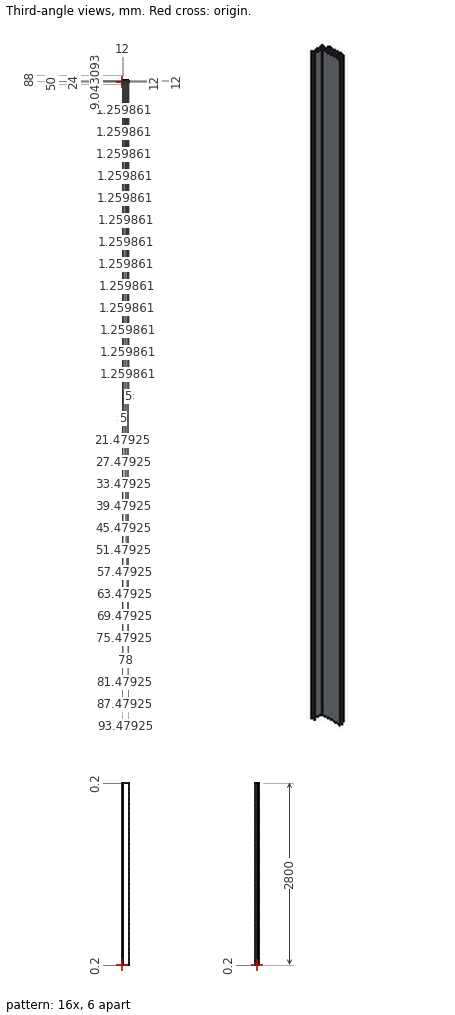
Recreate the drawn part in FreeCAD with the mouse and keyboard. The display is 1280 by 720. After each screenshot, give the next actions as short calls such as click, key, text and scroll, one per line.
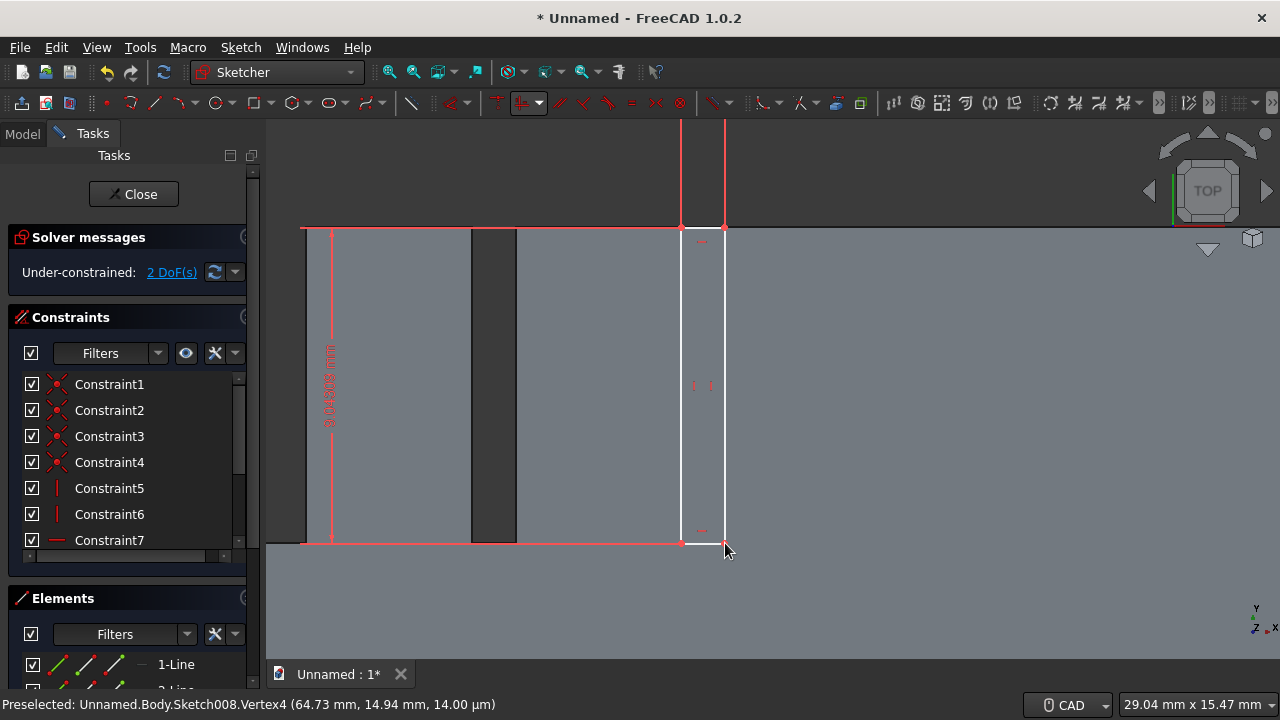
click(450, 104)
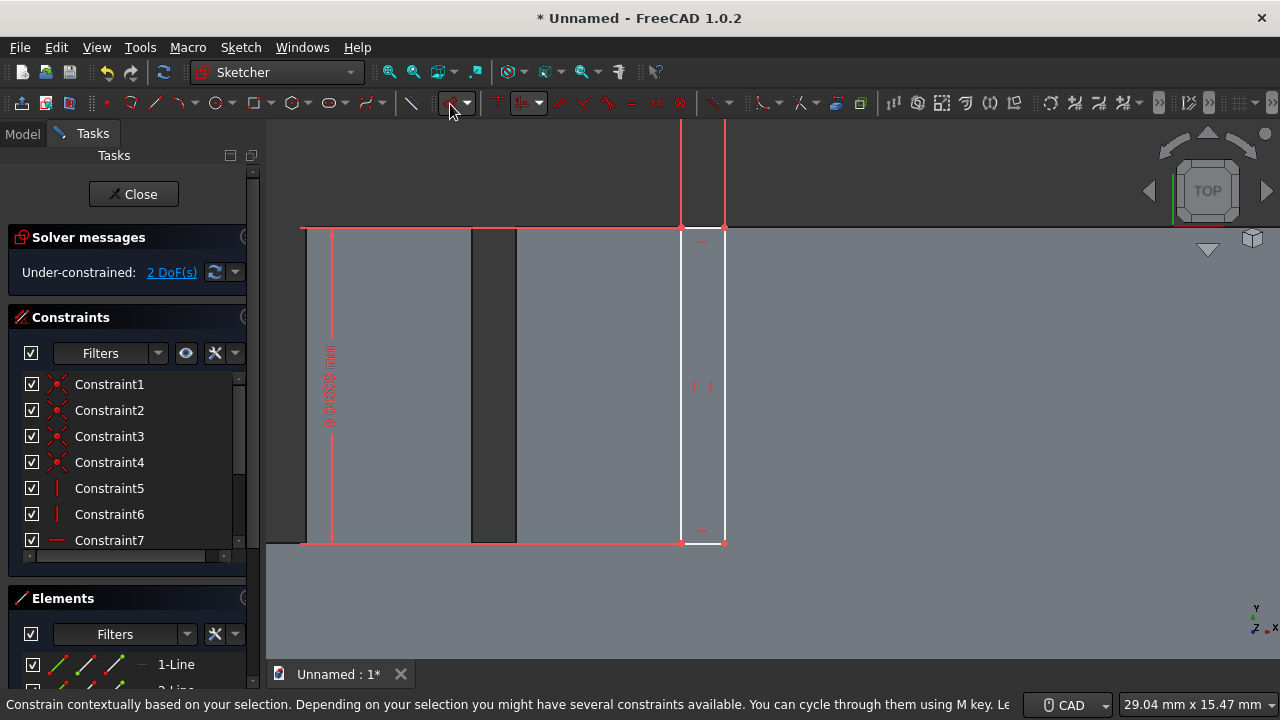
click(681, 228)
click(715, 571)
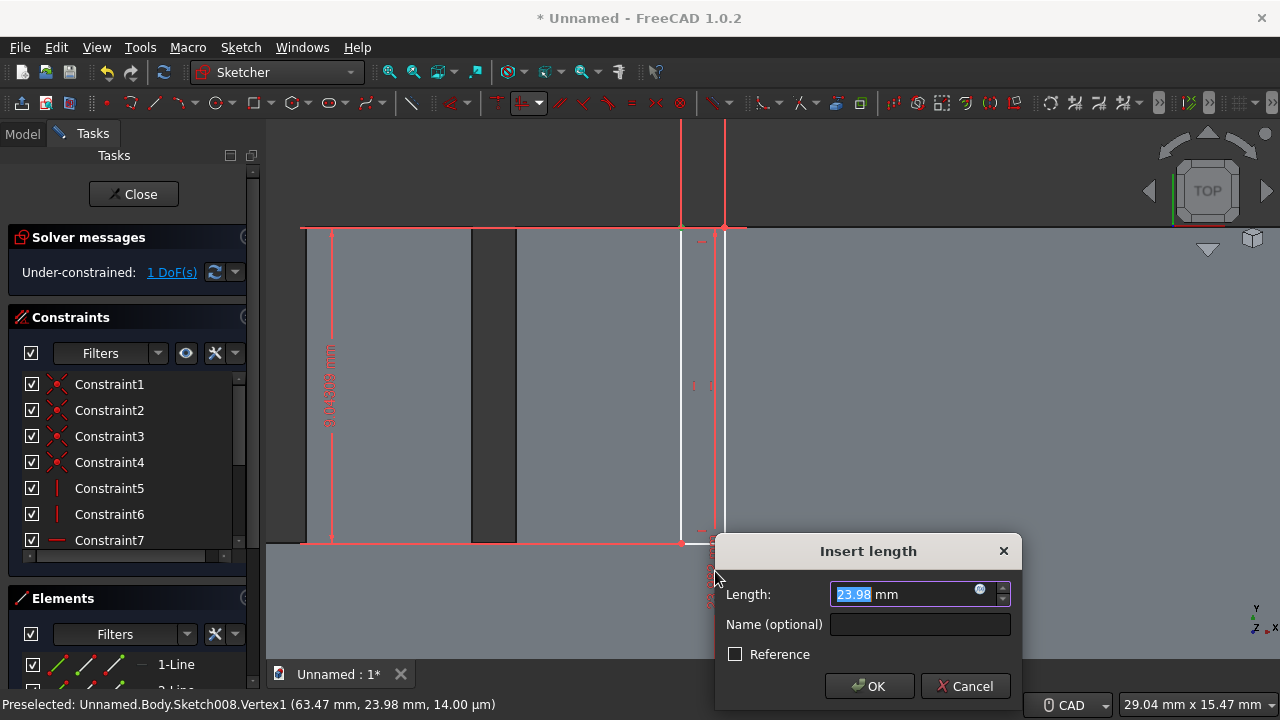
text(24)
key(Return)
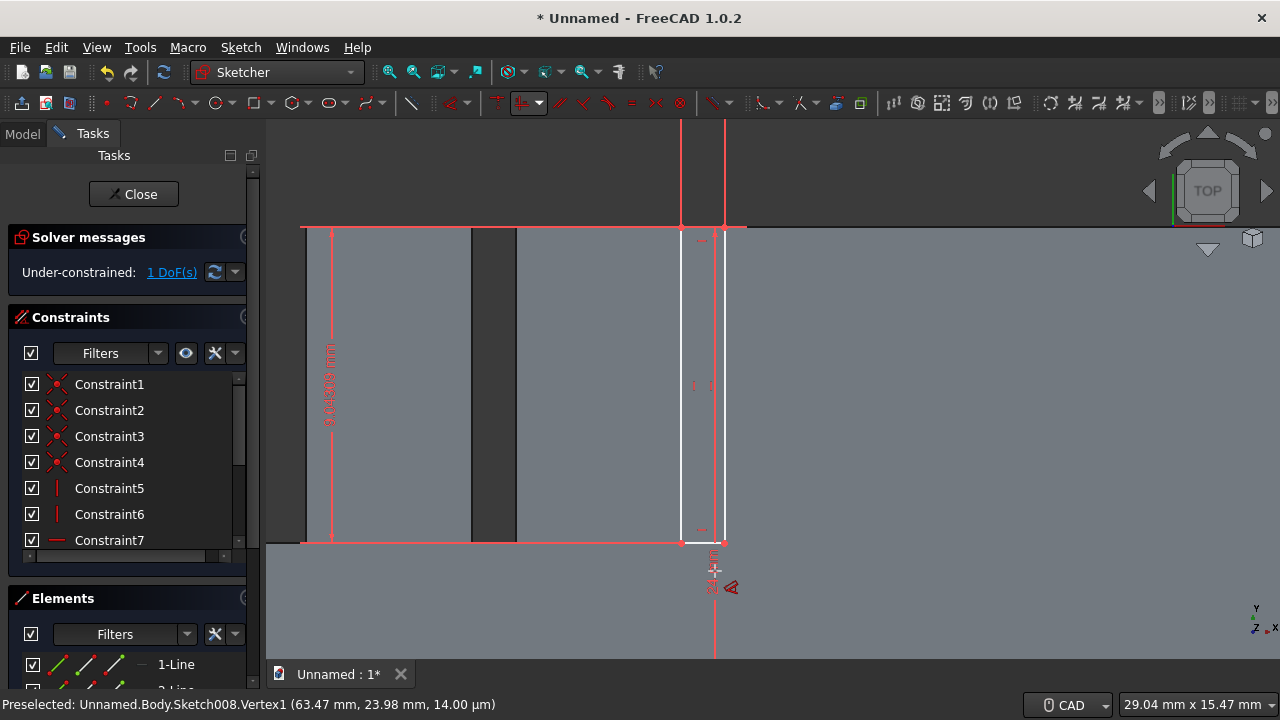
click(681, 227)
click(488, 193)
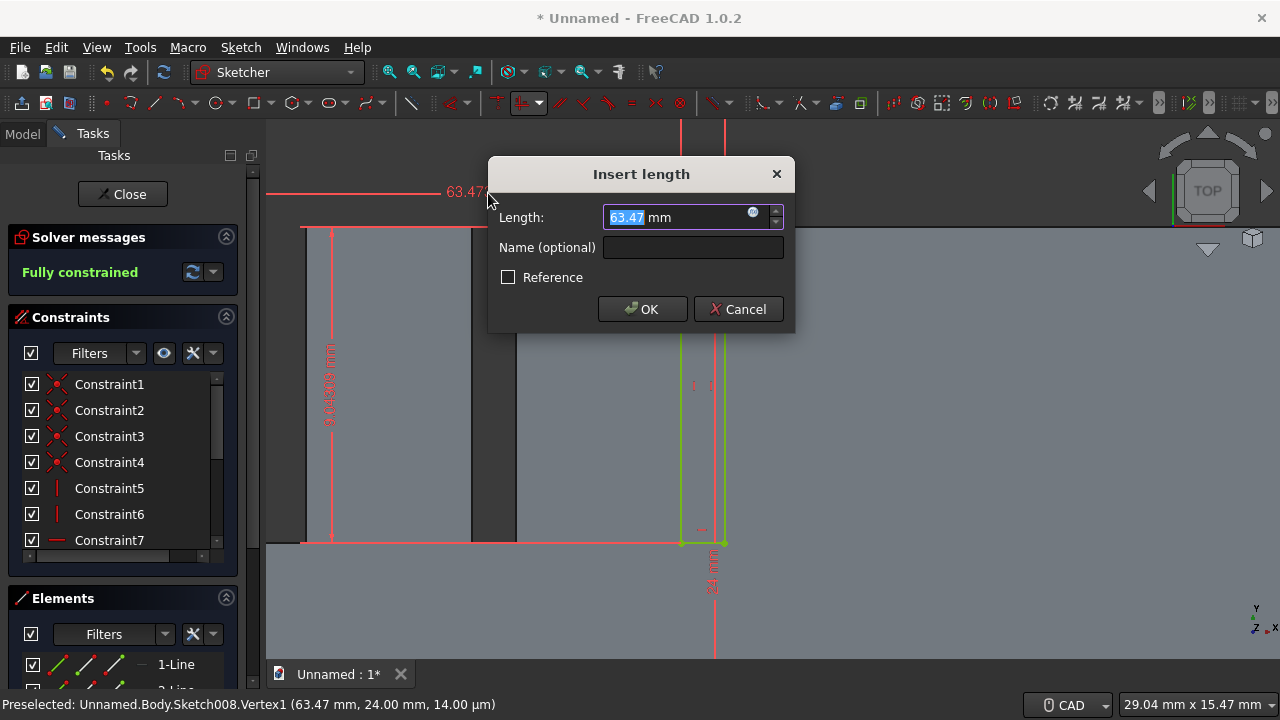
text(63.47925)
key(Return)
key(Escape)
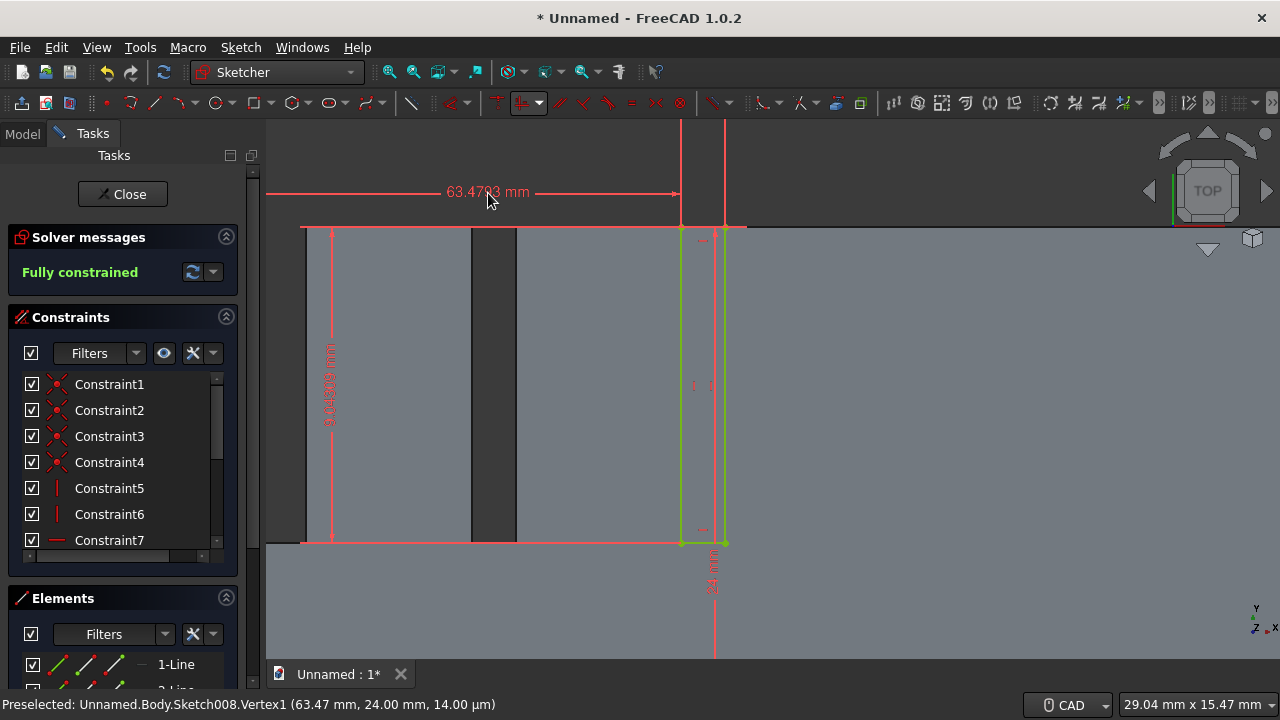
click(123, 194)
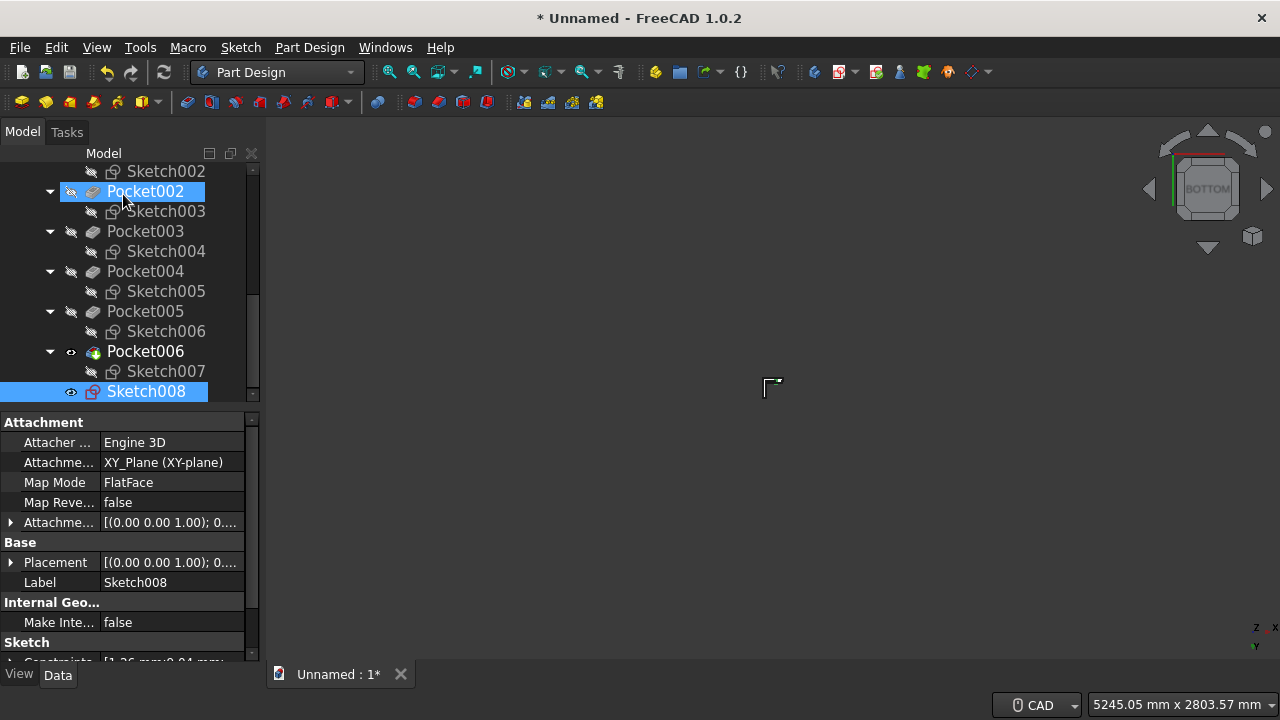
click(188, 102)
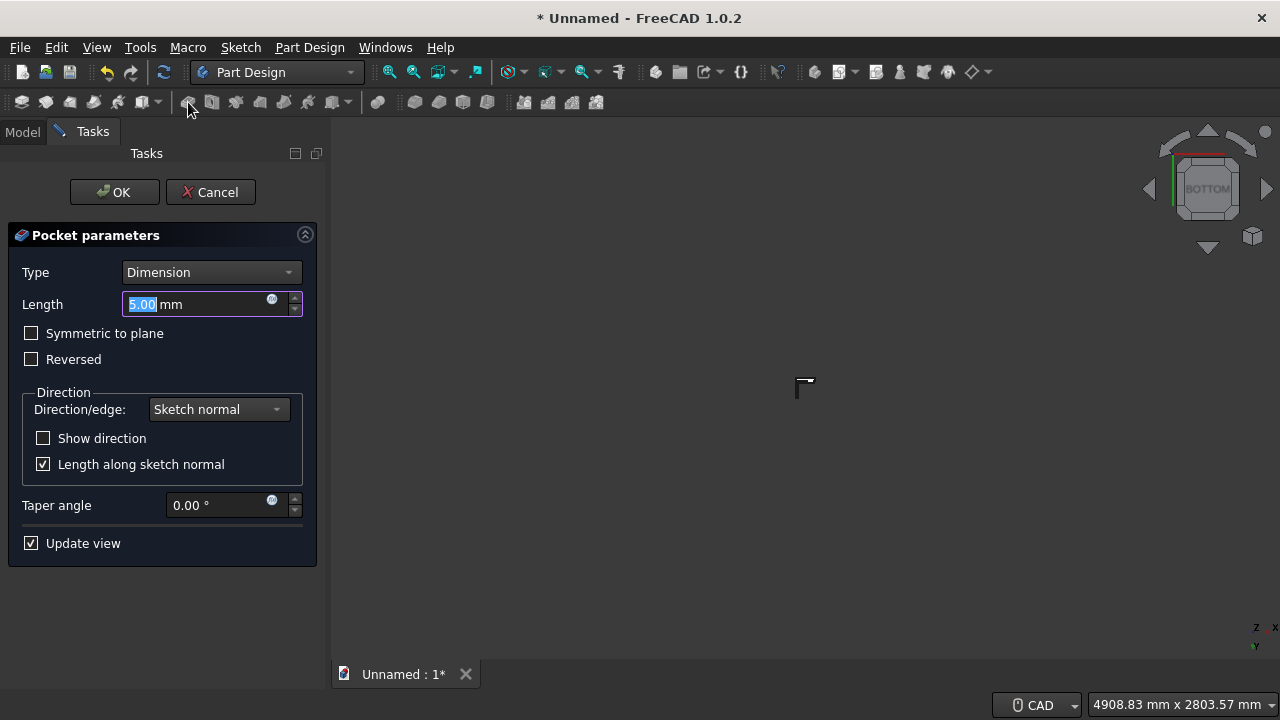
text(0.2)
key(Tab)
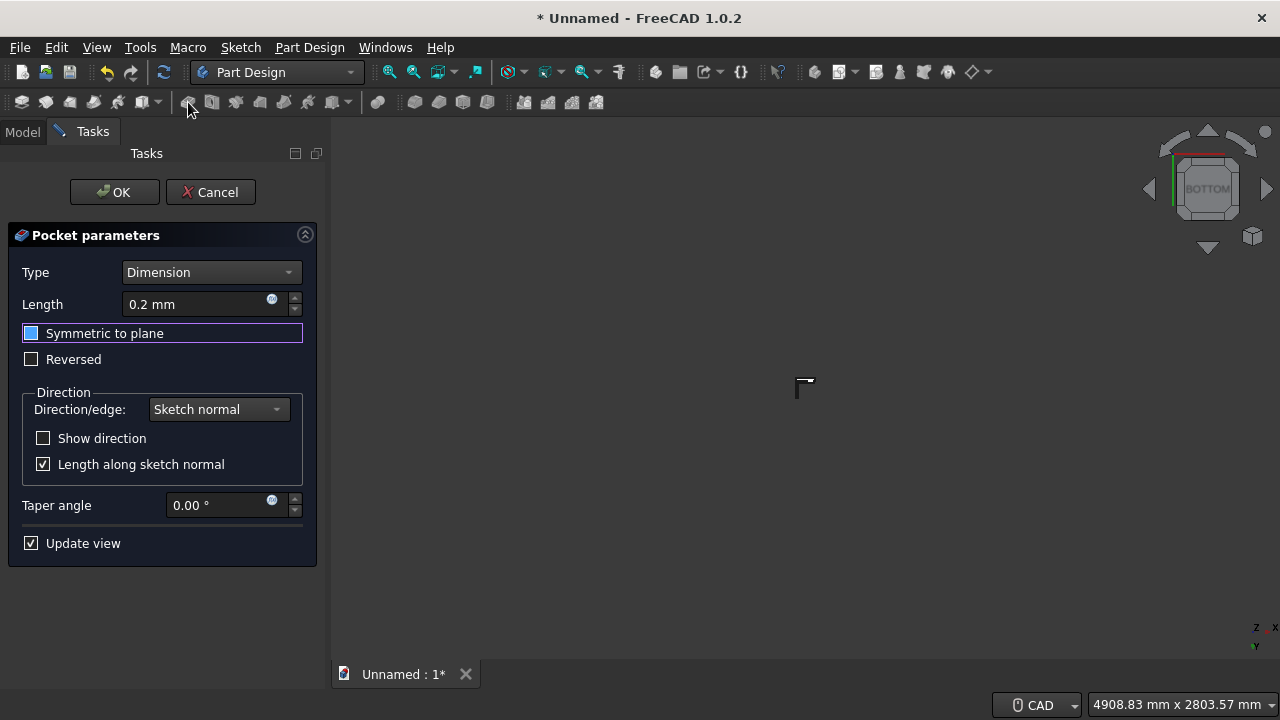
click(30, 359)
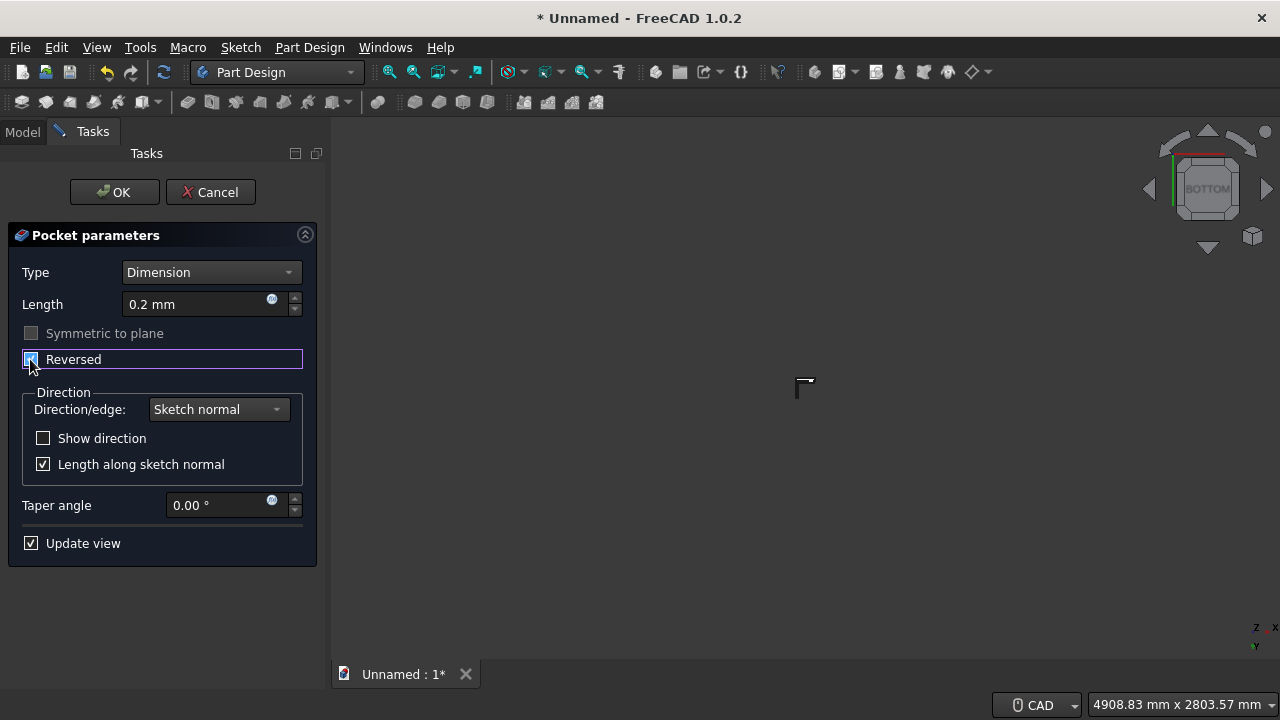
click(115, 192)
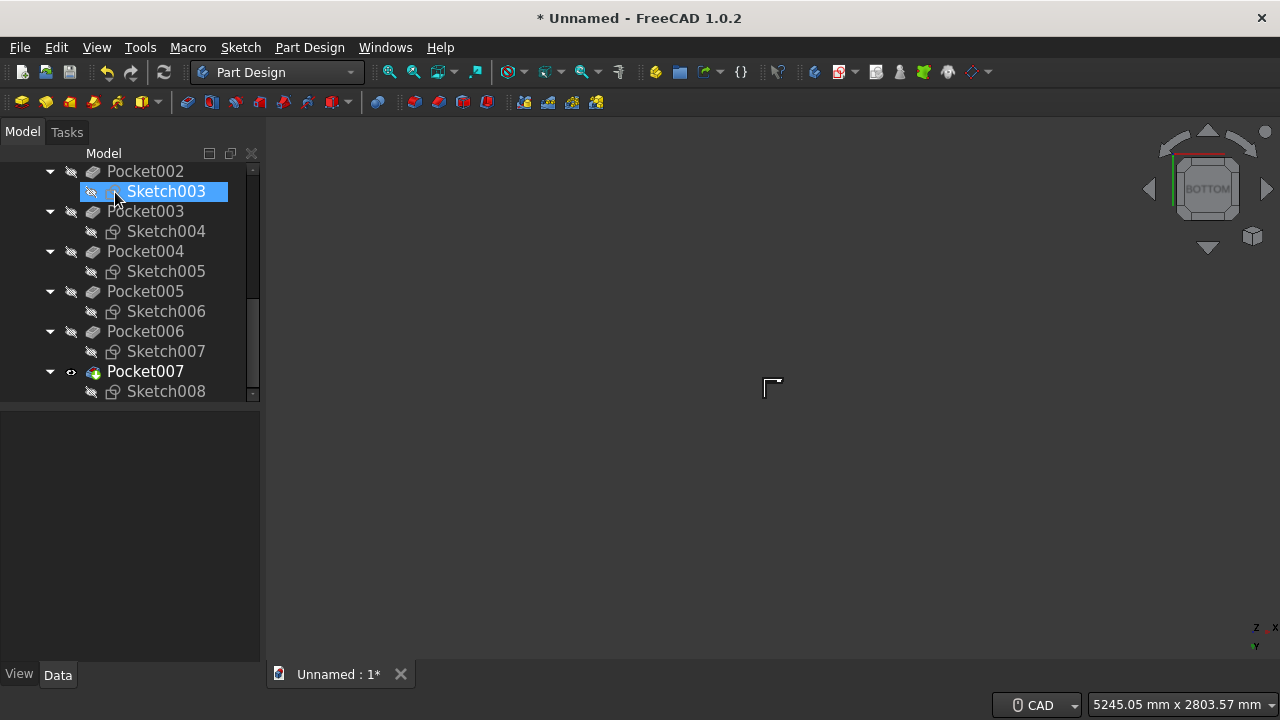
click(390, 72)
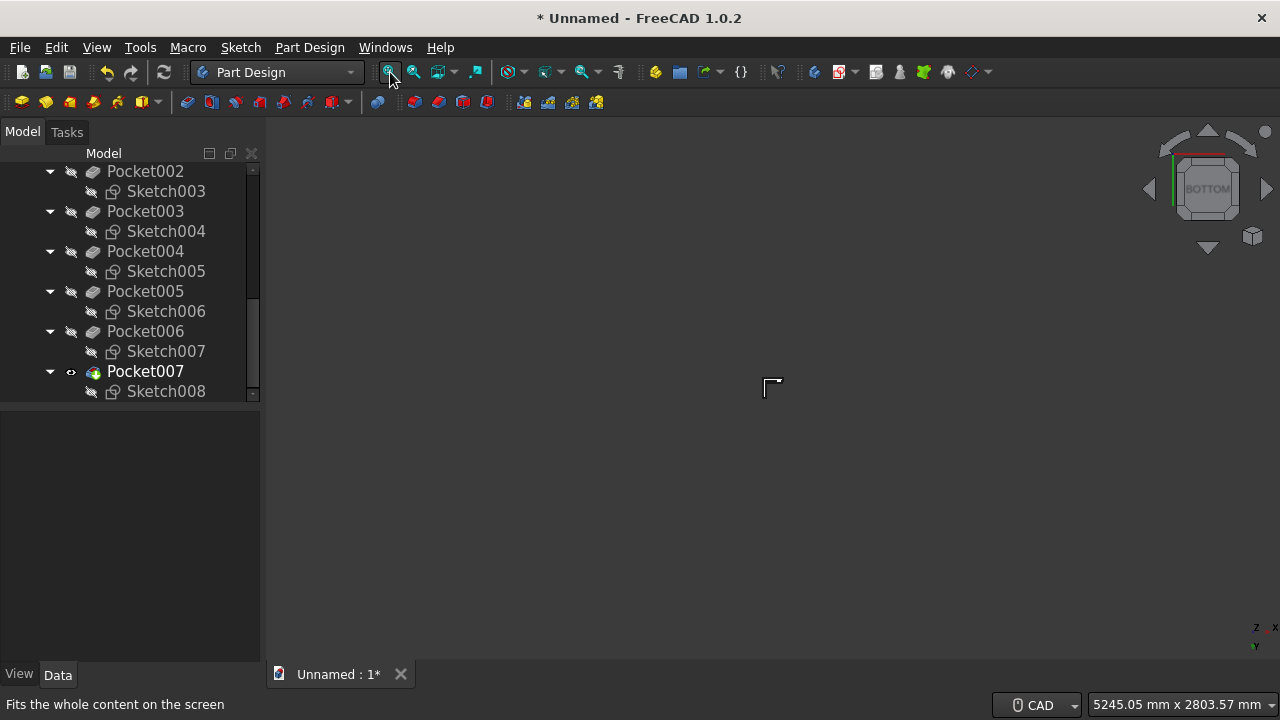
scroll(779, 379, up, 11)